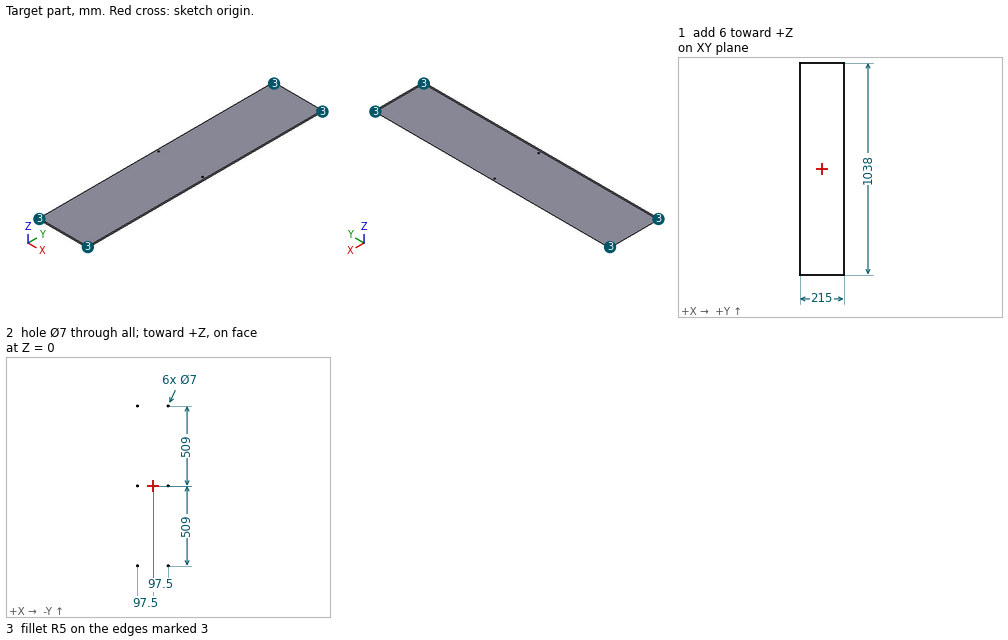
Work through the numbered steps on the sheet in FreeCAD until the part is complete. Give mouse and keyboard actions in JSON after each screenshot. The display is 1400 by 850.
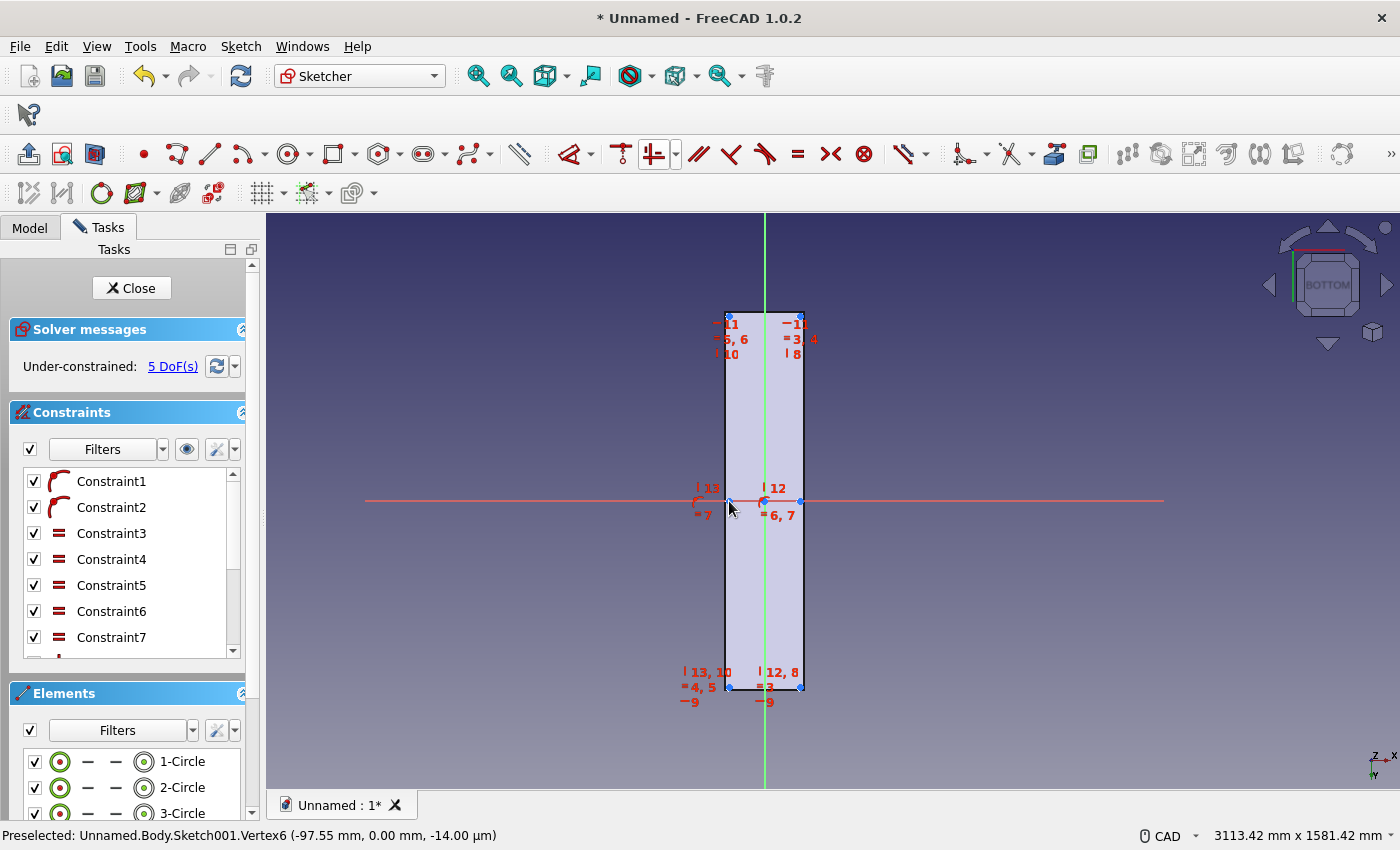
{"action": "scroll", "coordinate": [800, 685], "scroll_direction": "up", "scroll_amount": 14}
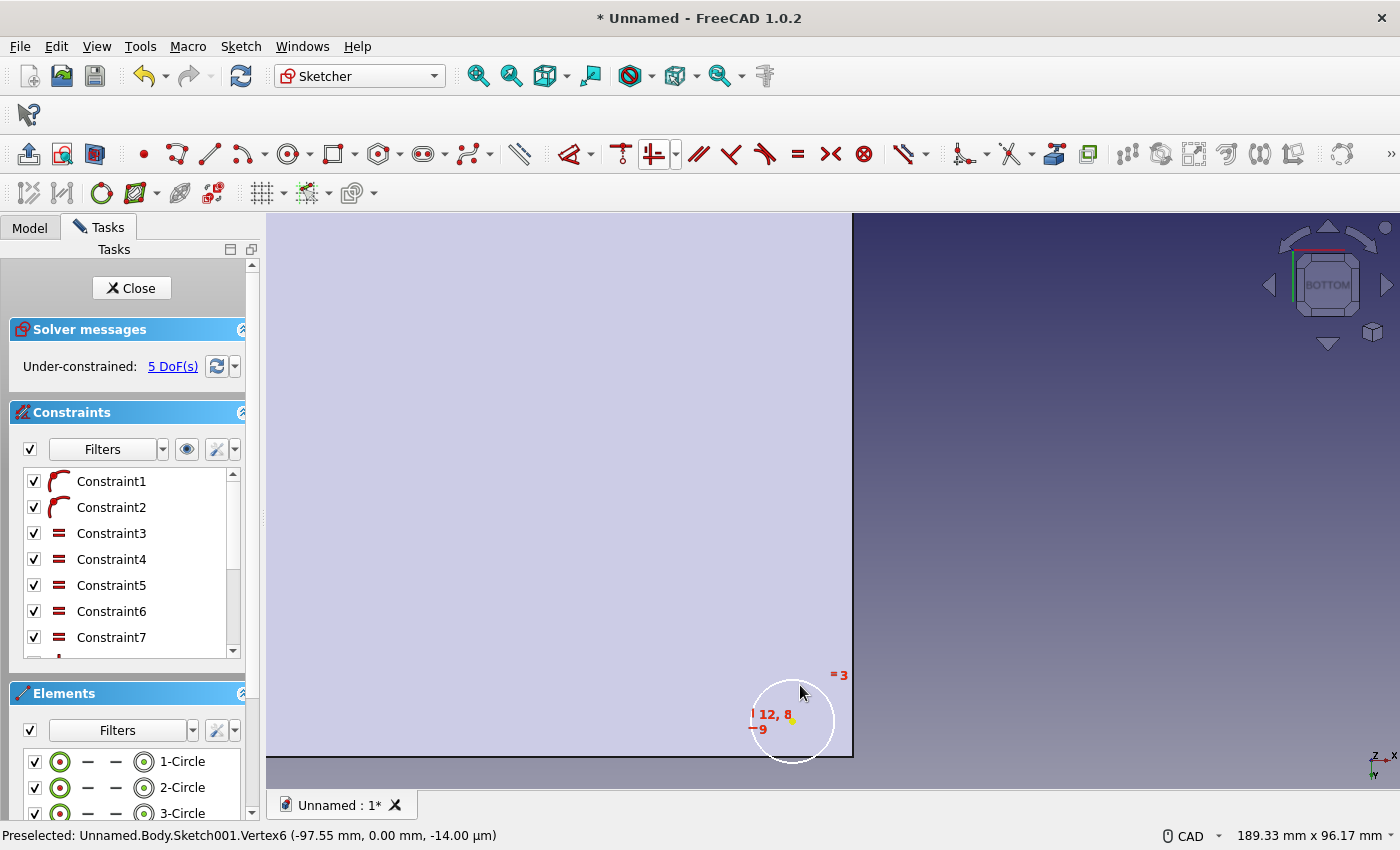
{"action": "left_click", "coordinate": [794, 680]}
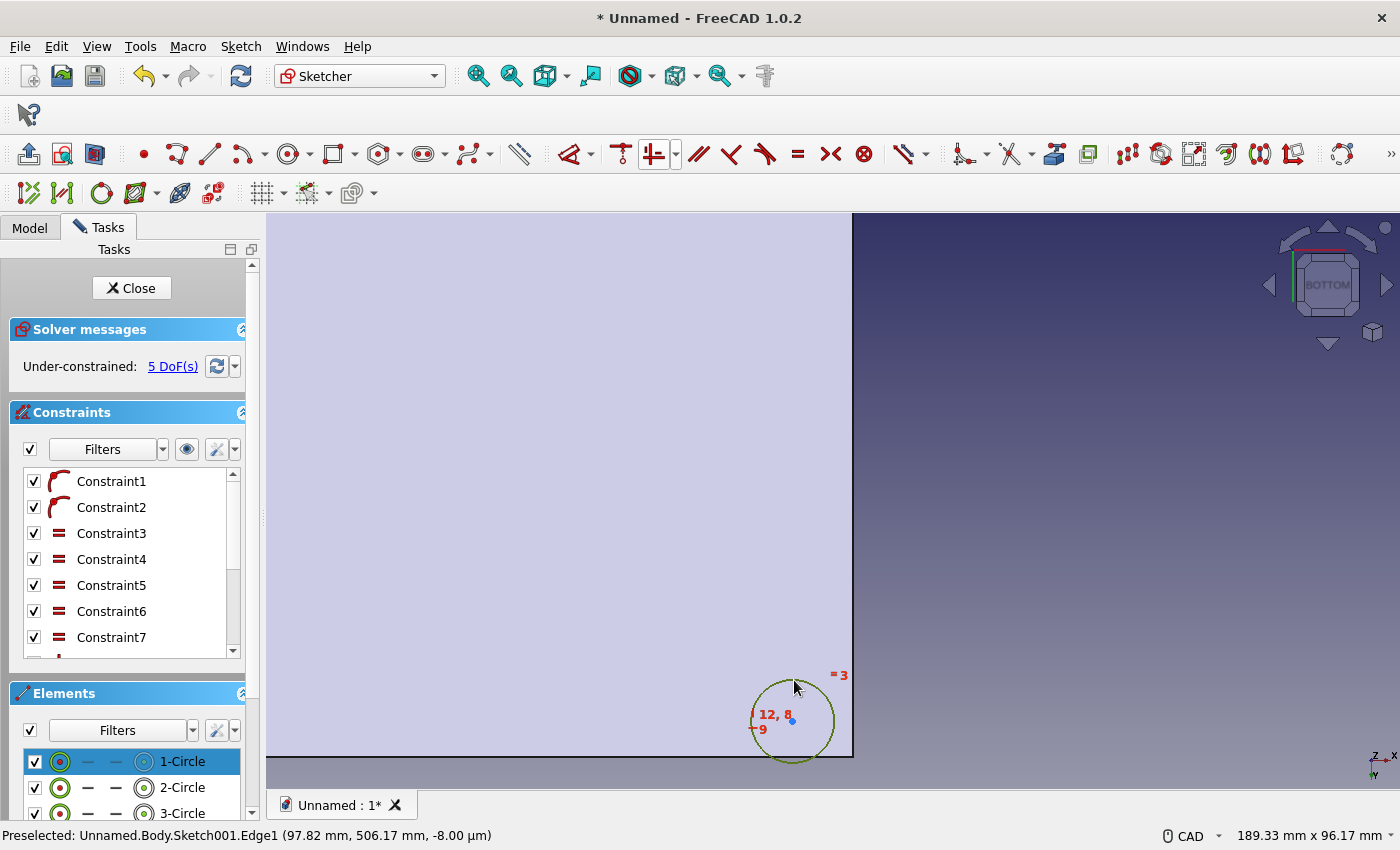
{"action": "key", "text": "k o"}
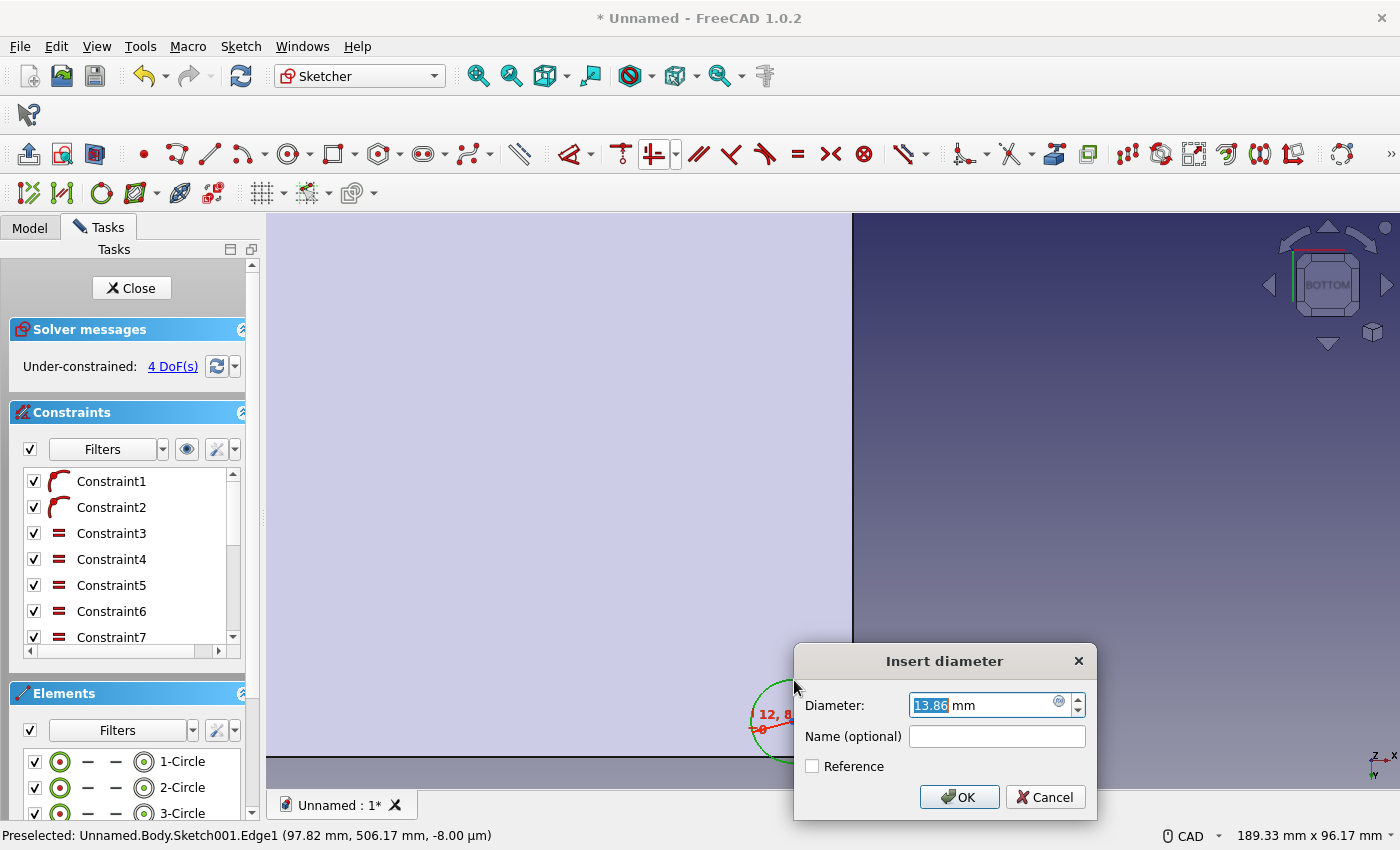
{"action": "type", "text": "7"}
{"action": "key", "text": "Return"}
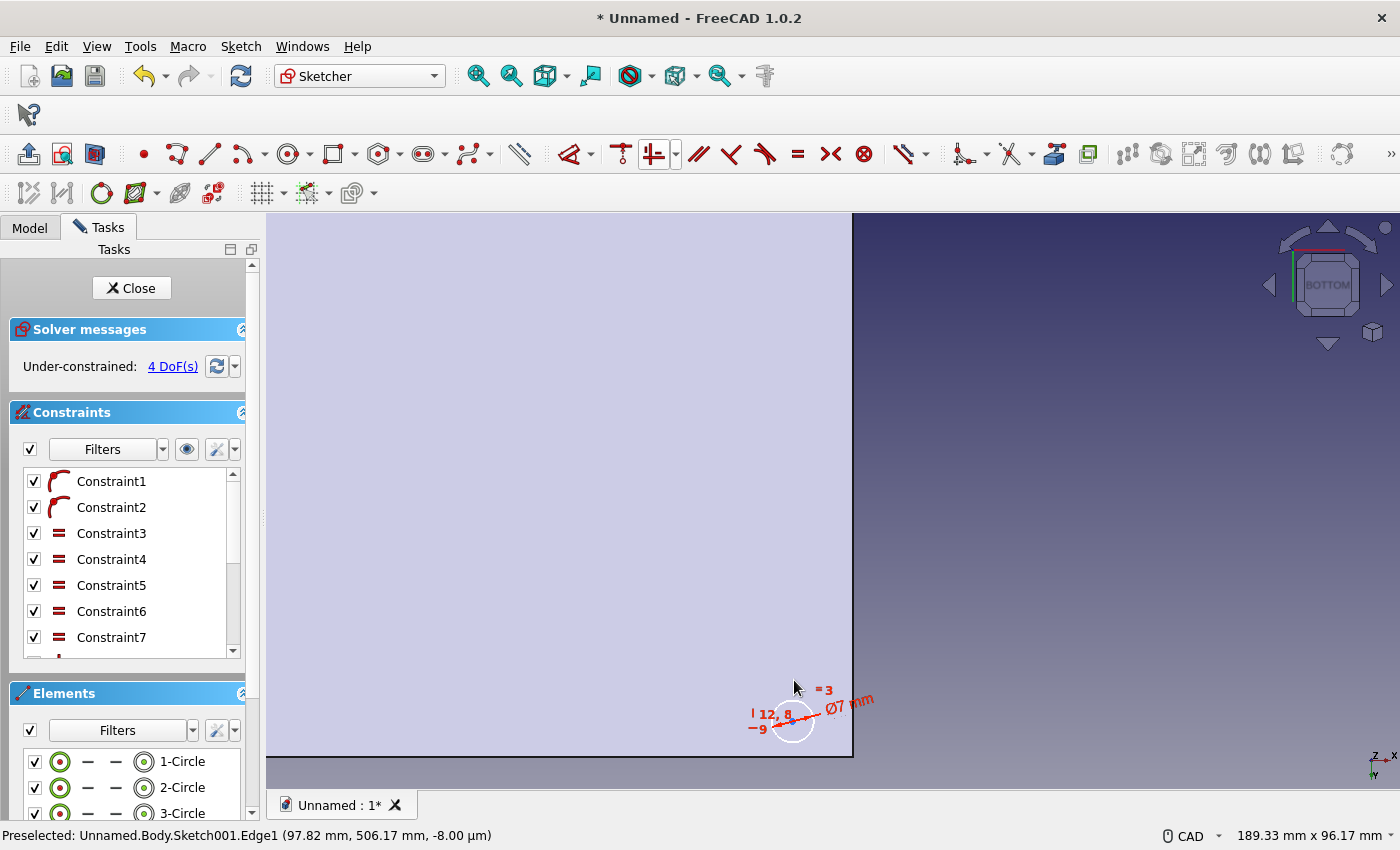
{"action": "scroll", "coordinate": [800, 686], "scroll_direction": "down", "scroll_amount": 14}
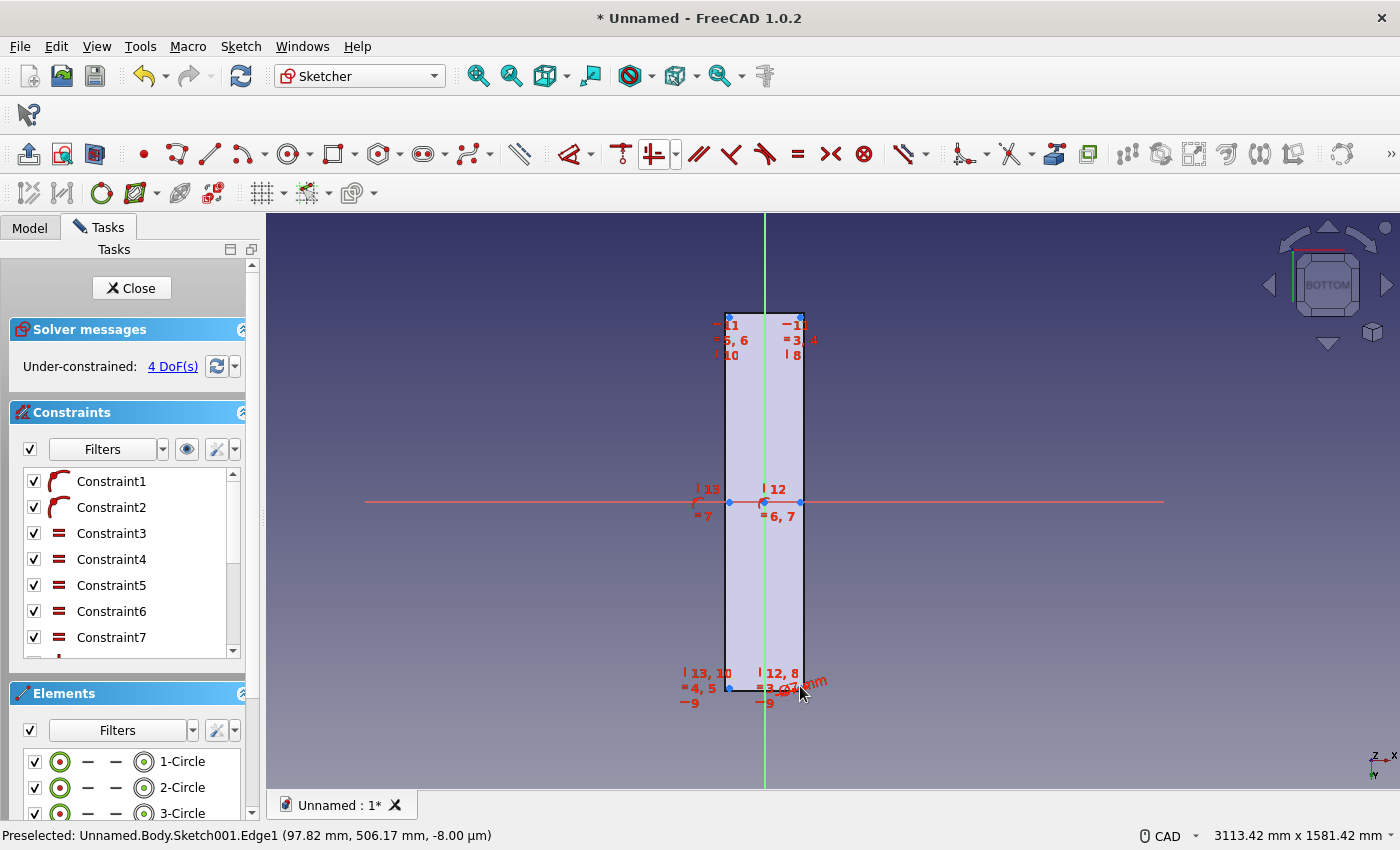
{"action": "left_click", "coordinate": [800, 689]}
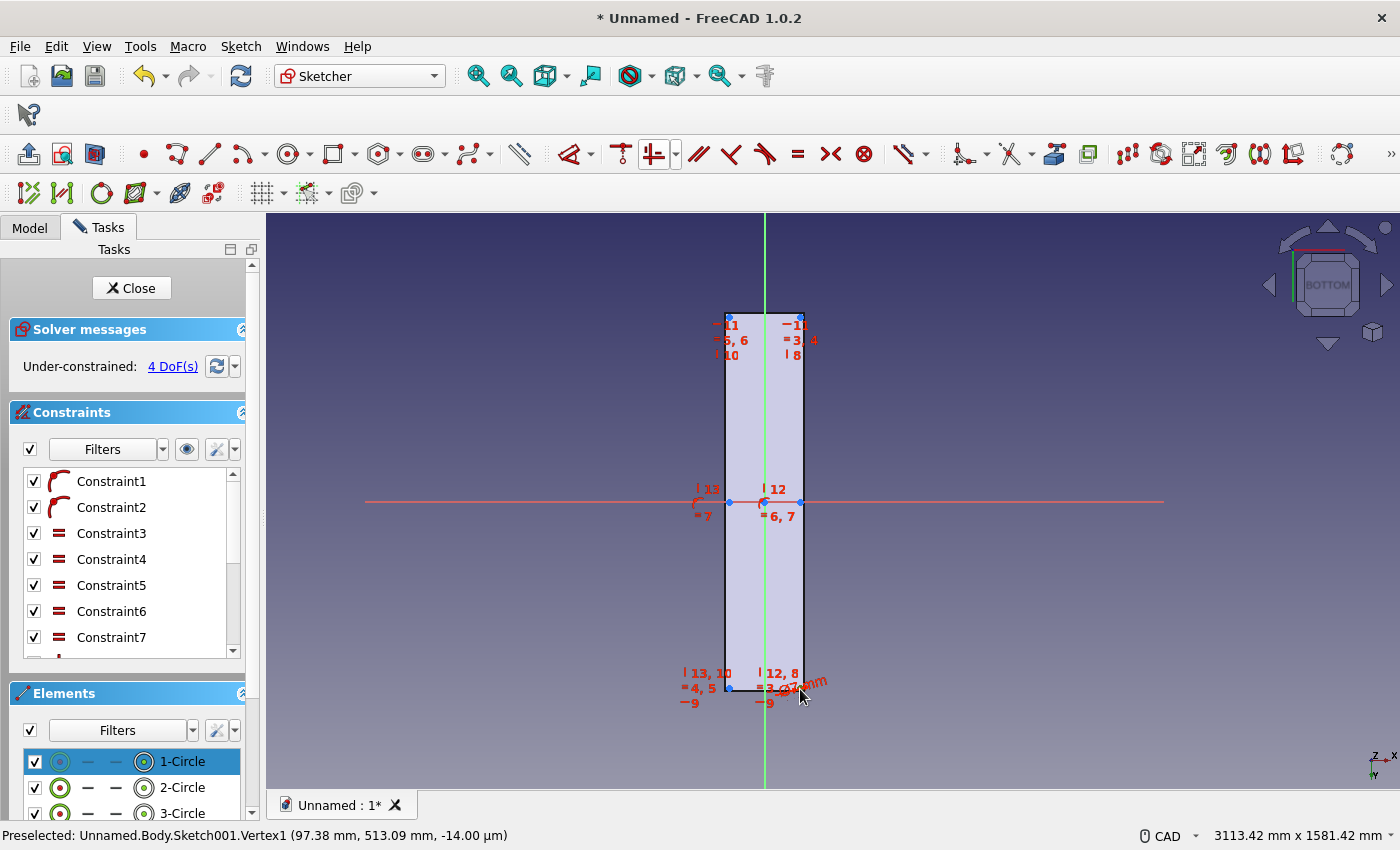
{"action": "left_click", "coordinate": [590, 154]}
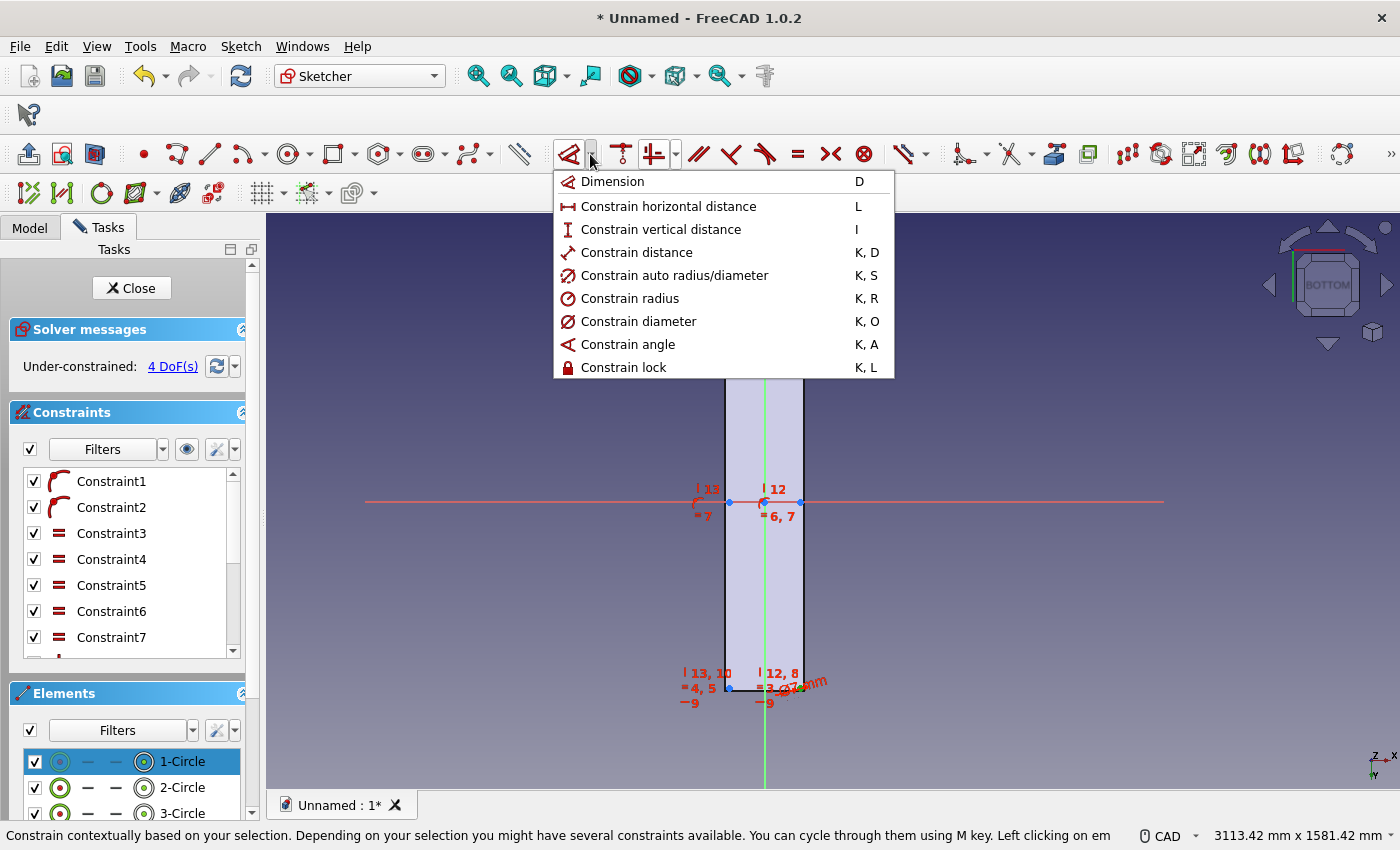
{"action": "left_click", "coordinate": [724, 230]}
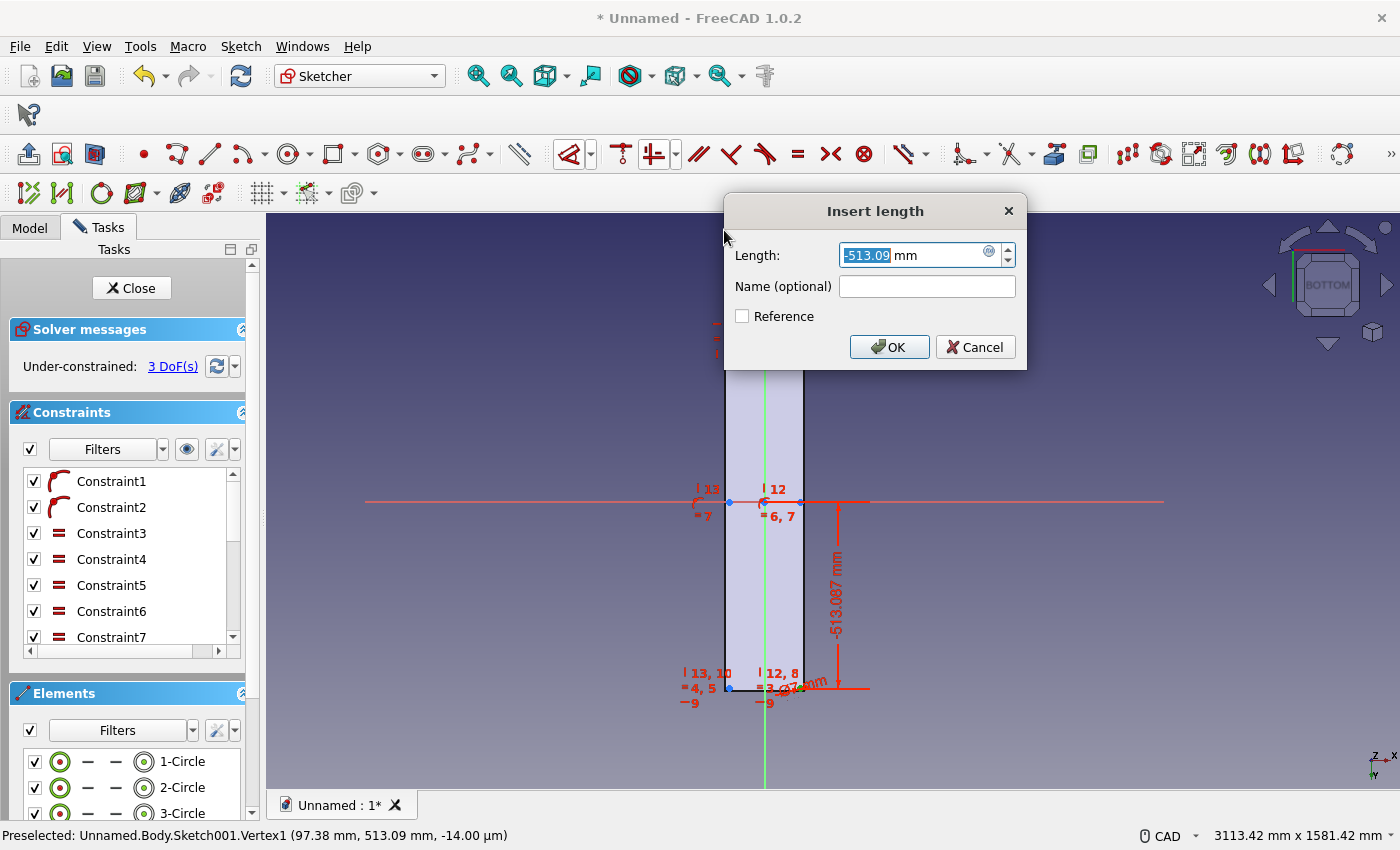
{"action": "type", "text": "-509"}
{"action": "key", "text": "Return"}